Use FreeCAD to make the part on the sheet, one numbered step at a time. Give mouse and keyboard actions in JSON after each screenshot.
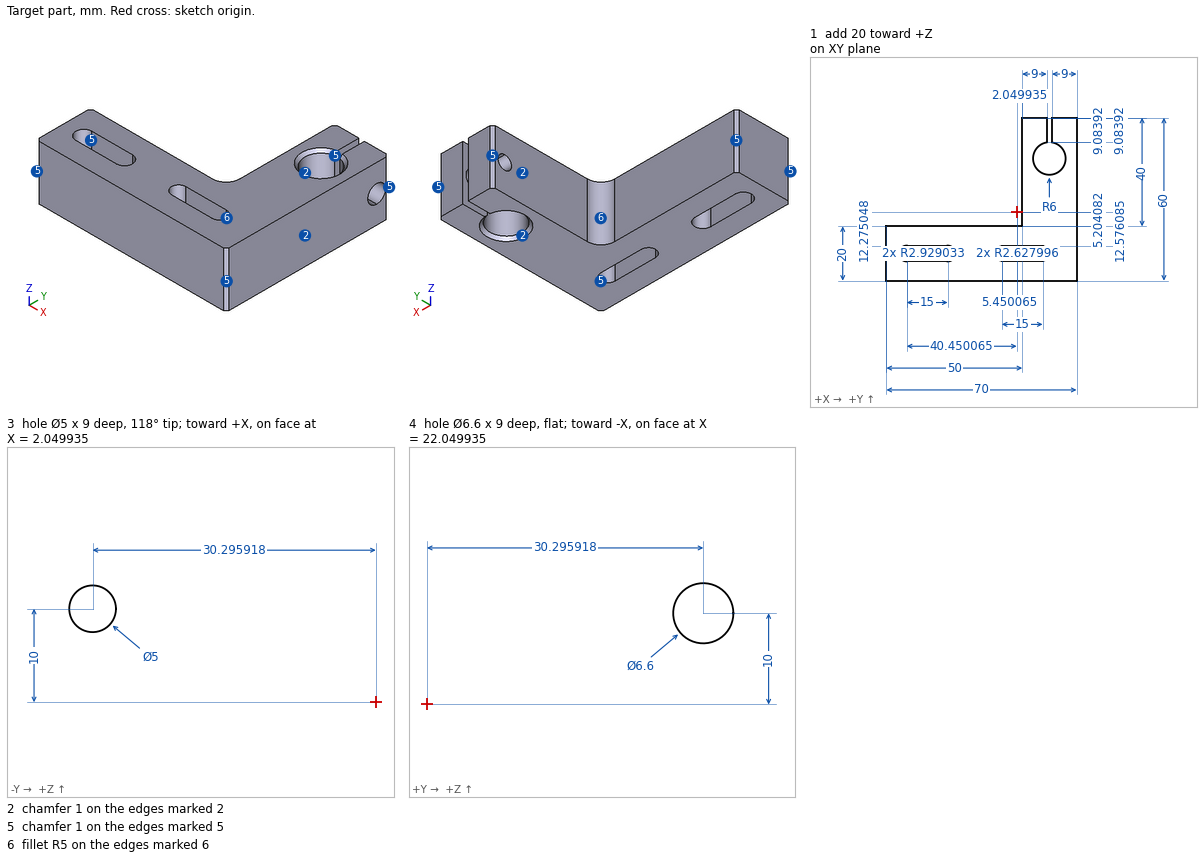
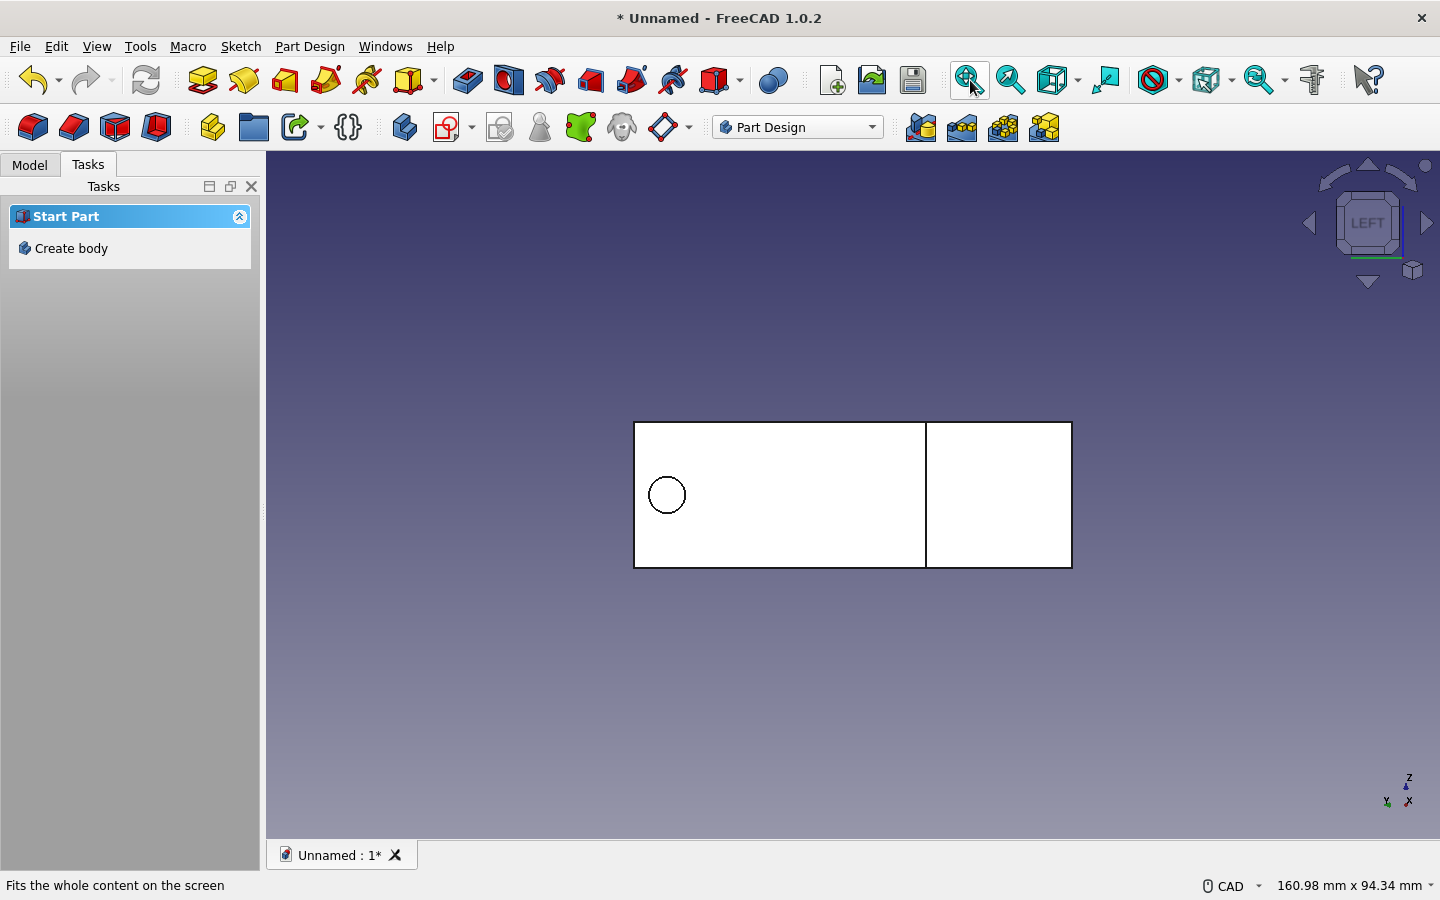
{"action": "key", "text": "0"}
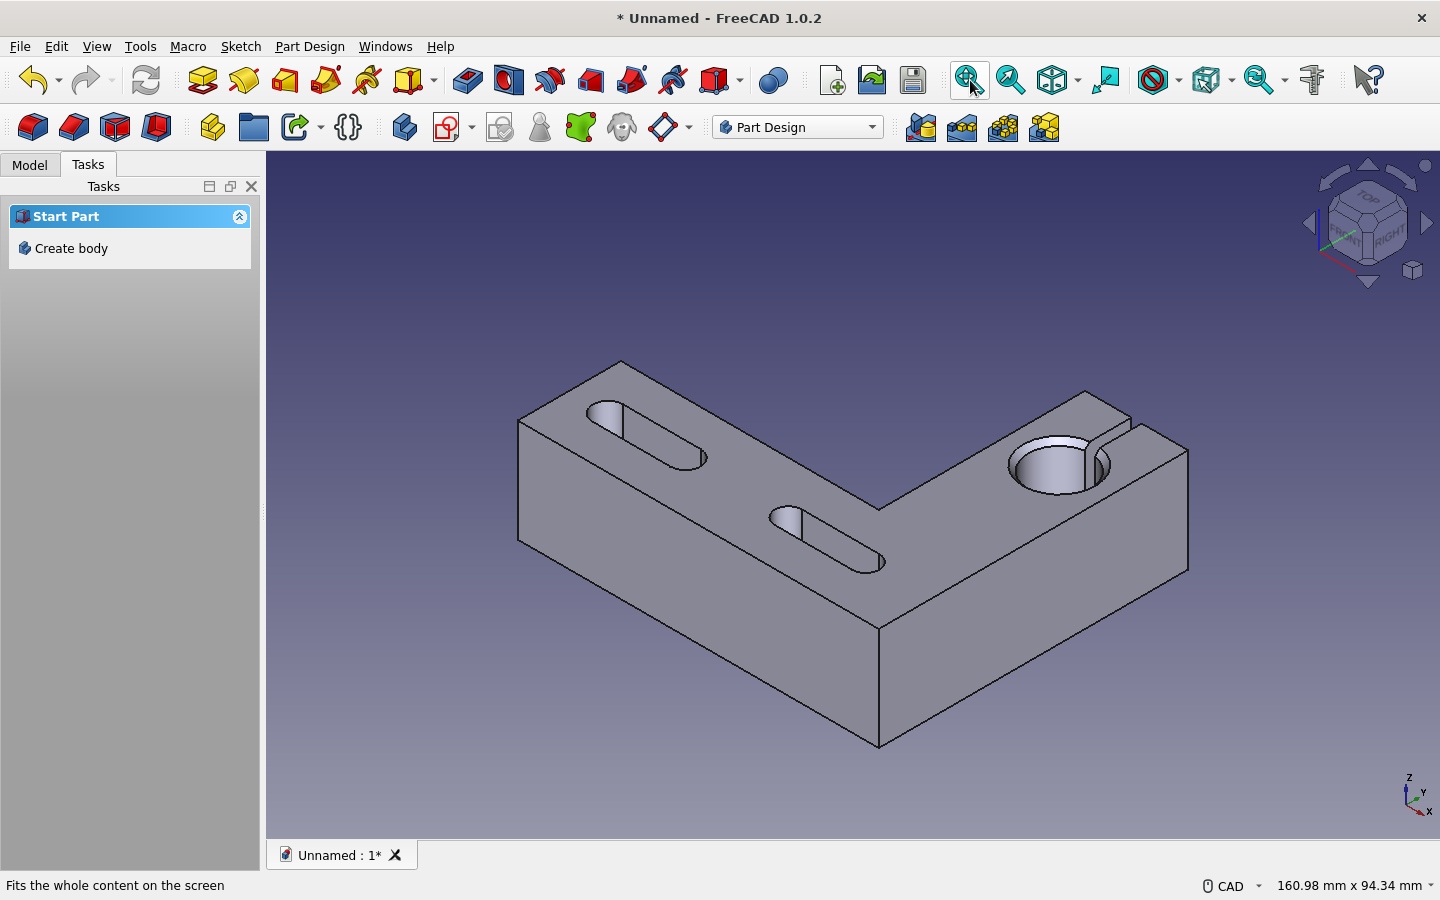
{"action": "left_click", "coordinate": [1122, 547]}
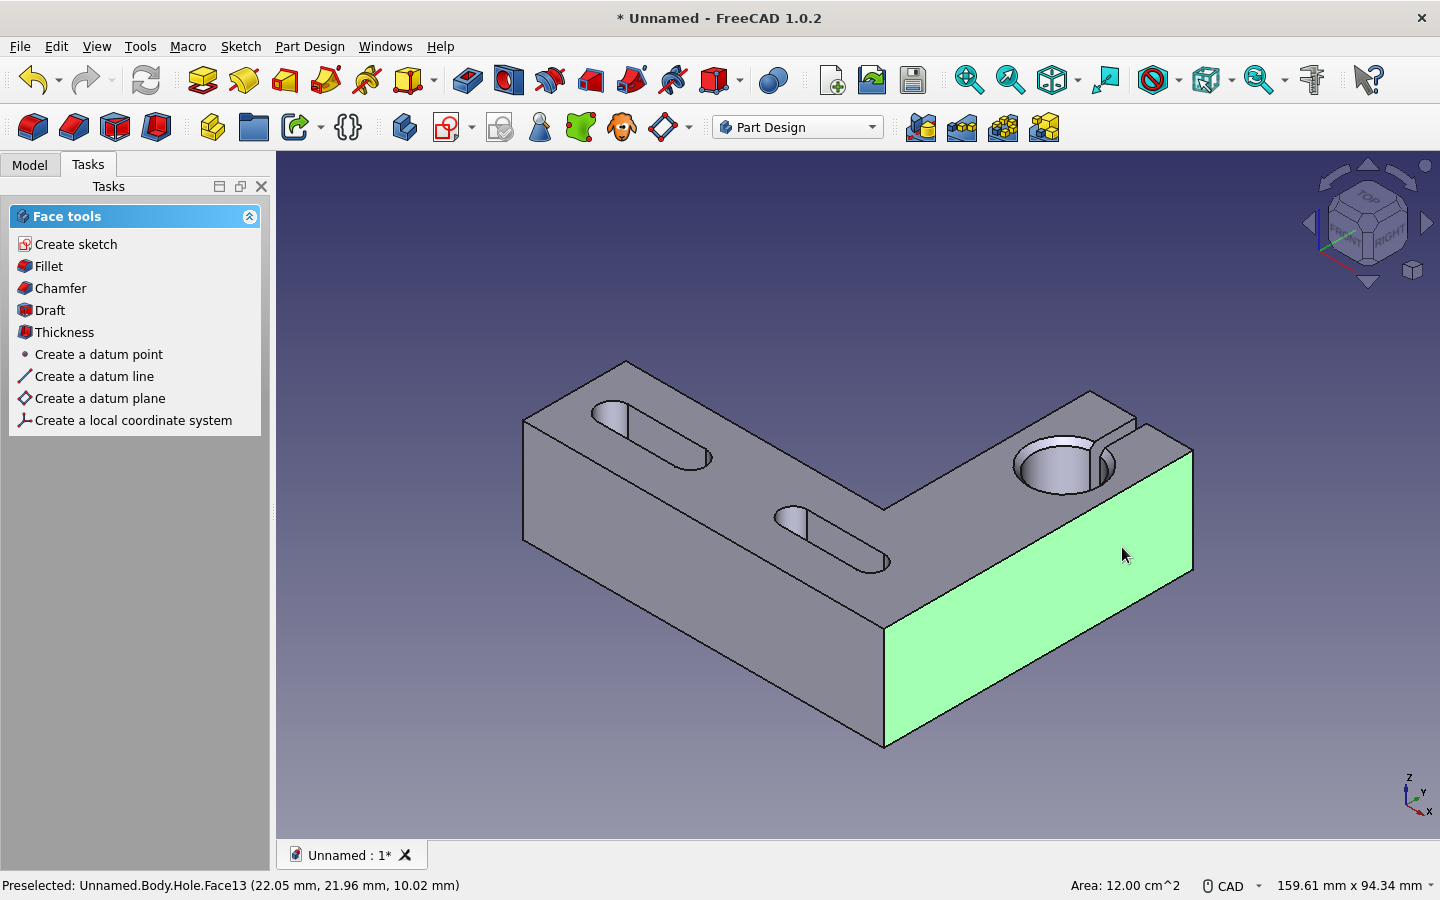
{"action": "left_click", "coordinate": [446, 128]}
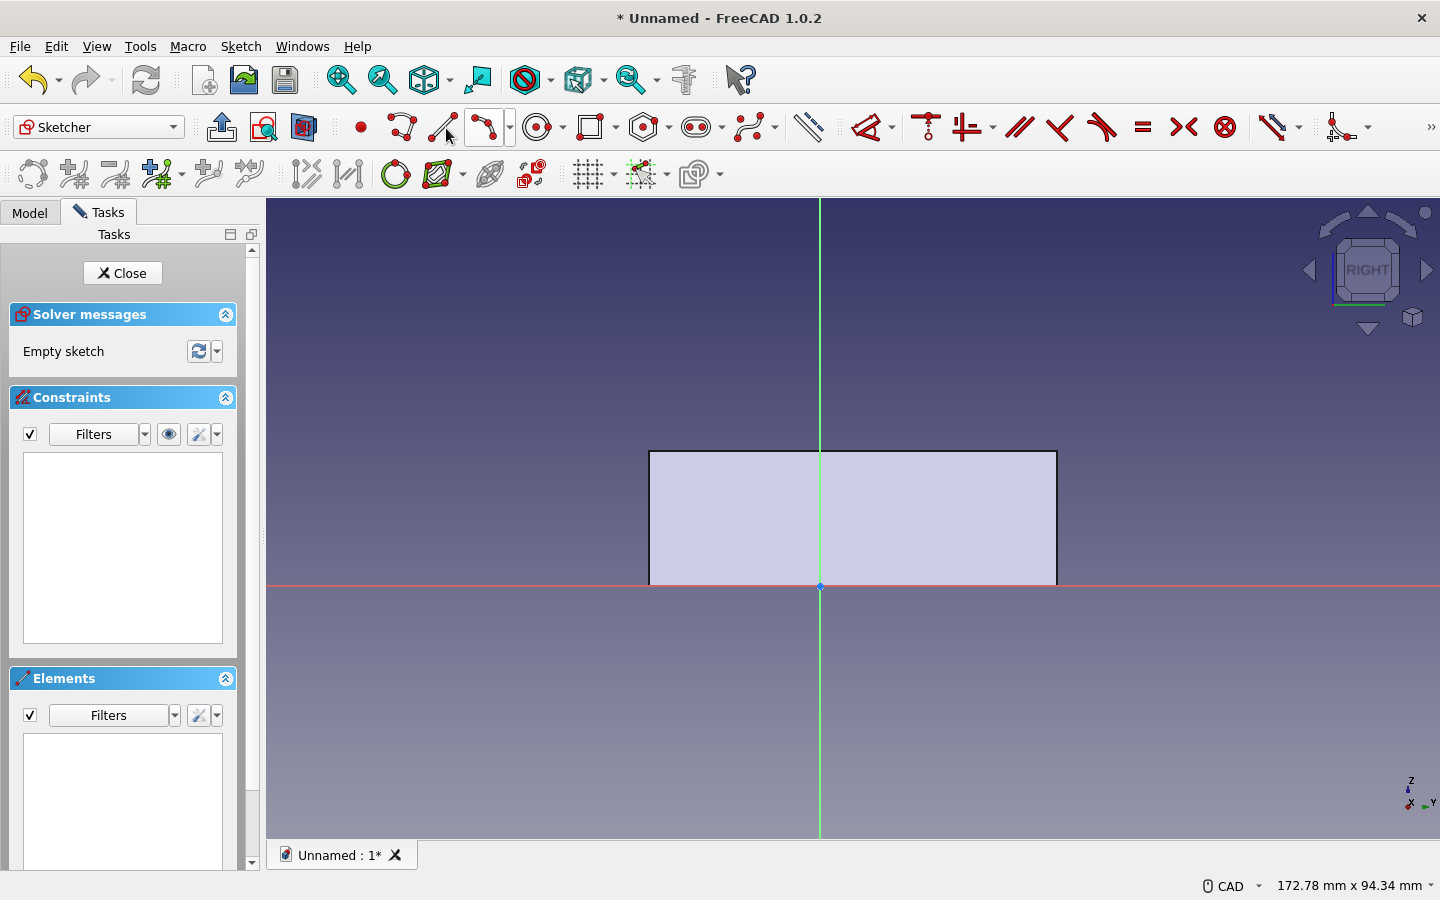
{"action": "scroll", "coordinate": [1056, 518], "scroll_direction": "up", "scroll_amount": 11}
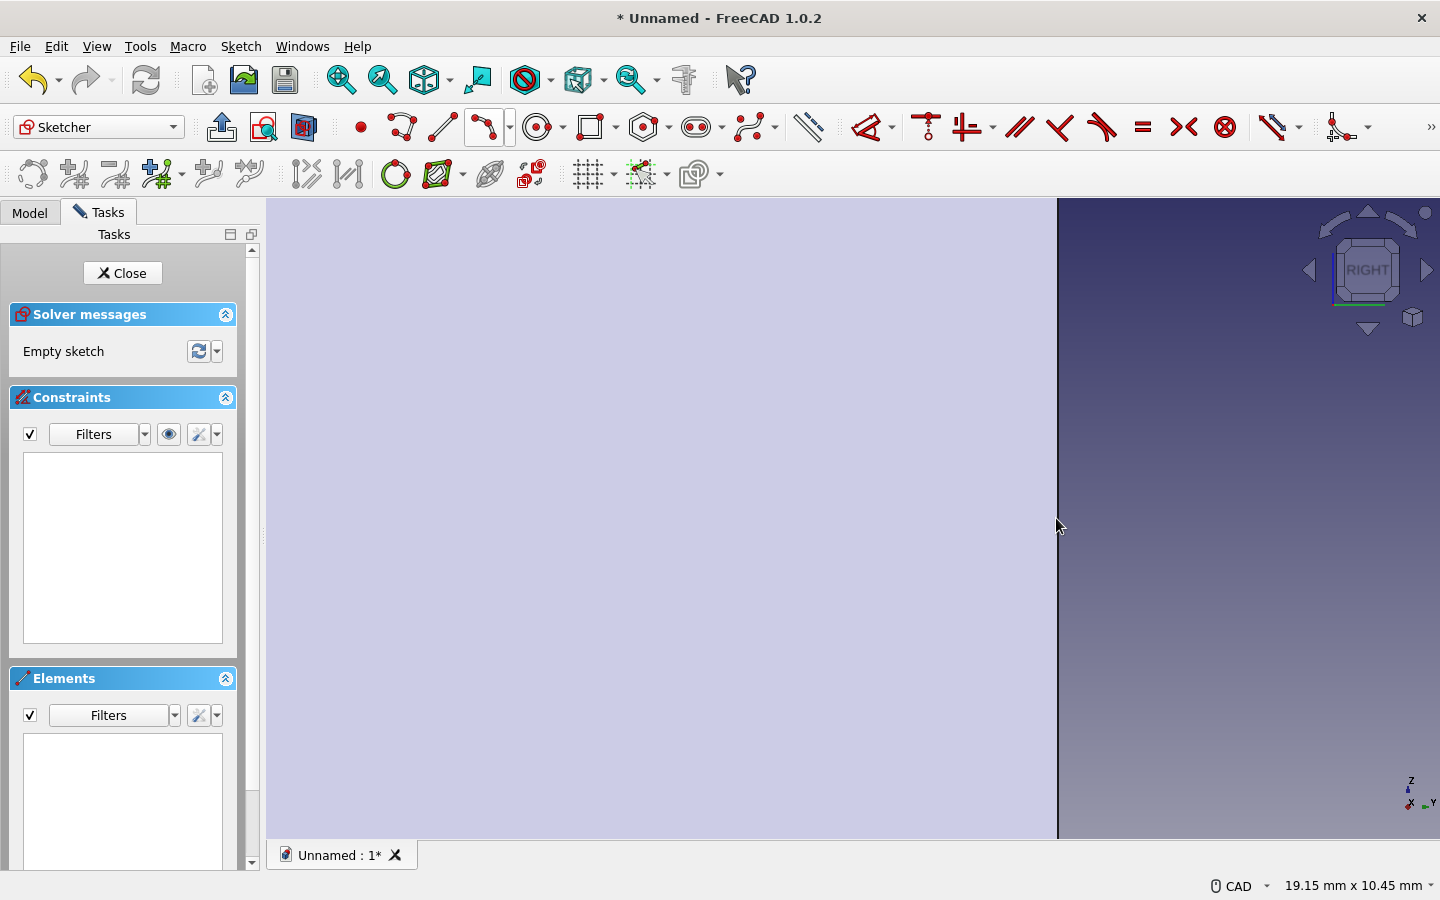
{"action": "left_click", "coordinate": [536, 128]}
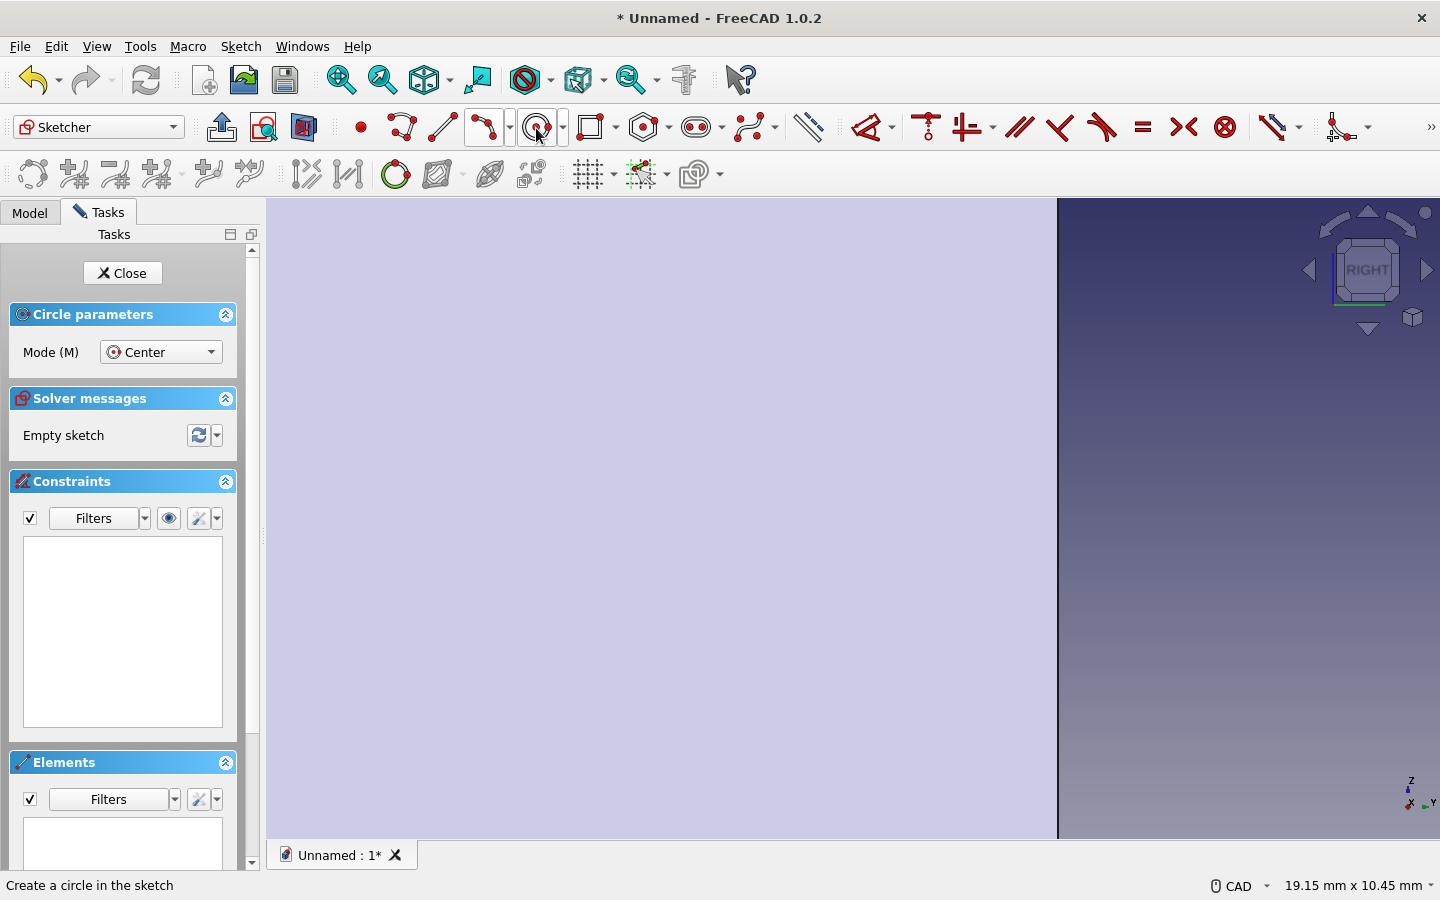
{"action": "left_click", "coordinate": [782, 518]}
{"action": "left_click", "coordinate": [925, 375]}
{"action": "key", "text": "Escape"}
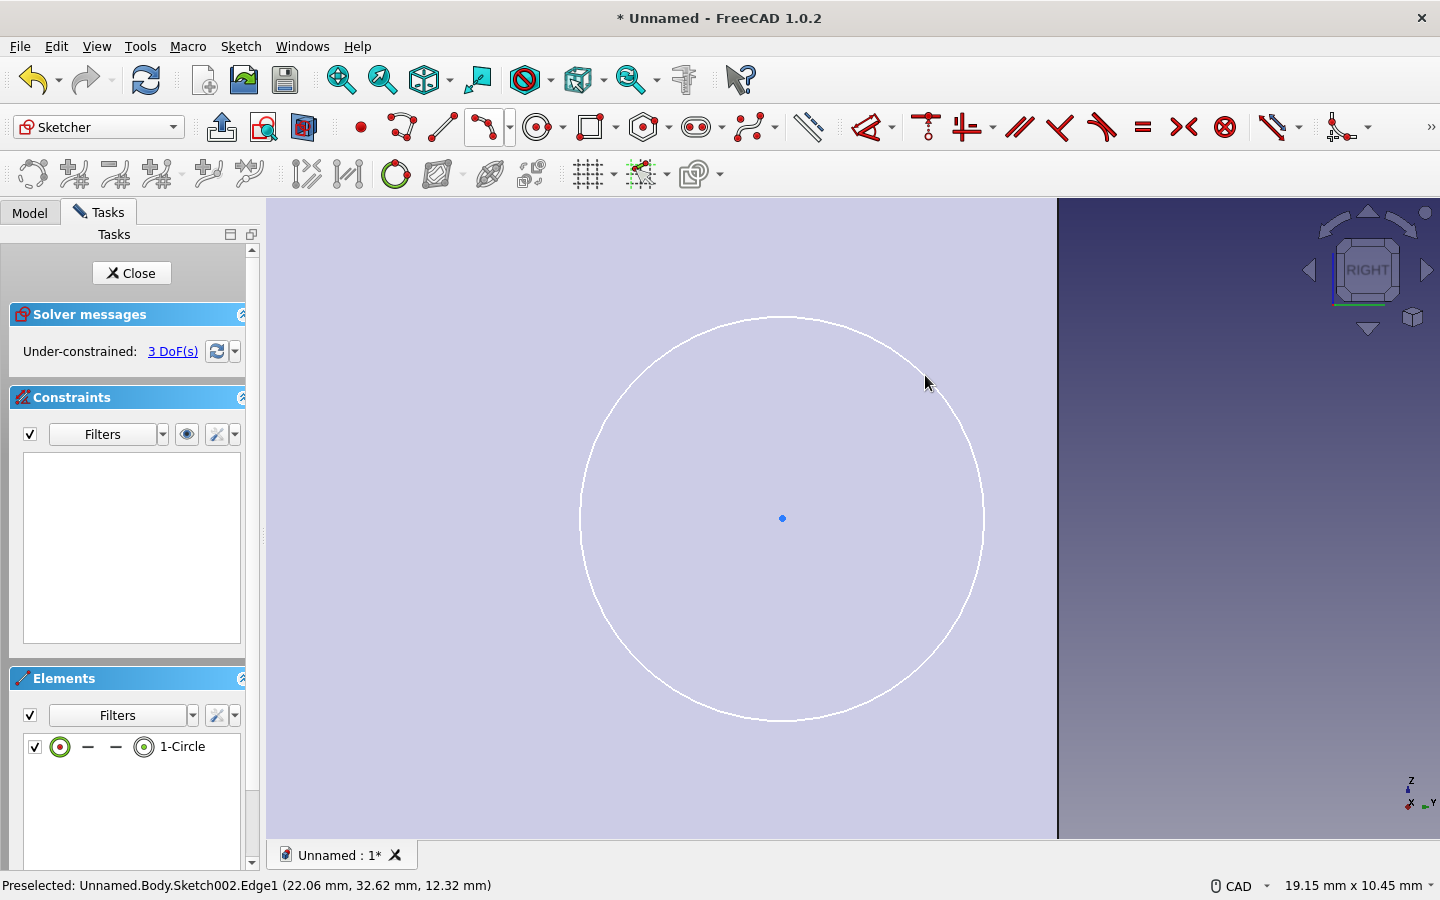
{"action": "left_click", "coordinate": [866, 128]}